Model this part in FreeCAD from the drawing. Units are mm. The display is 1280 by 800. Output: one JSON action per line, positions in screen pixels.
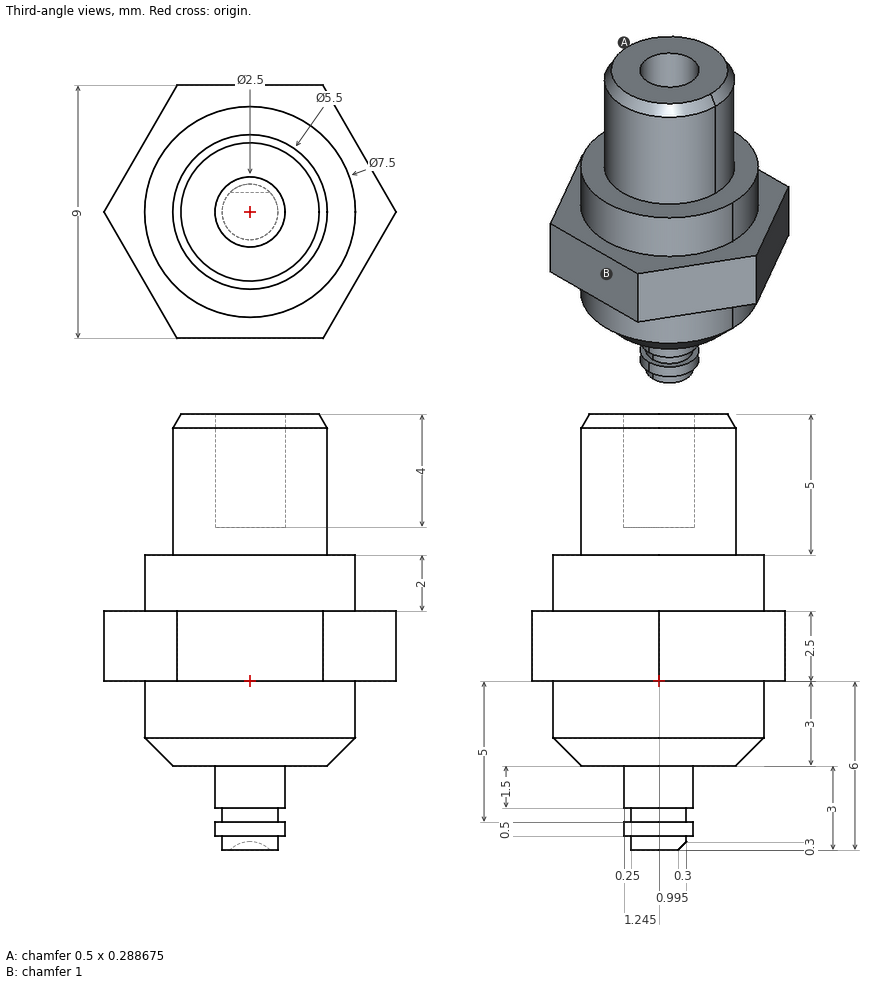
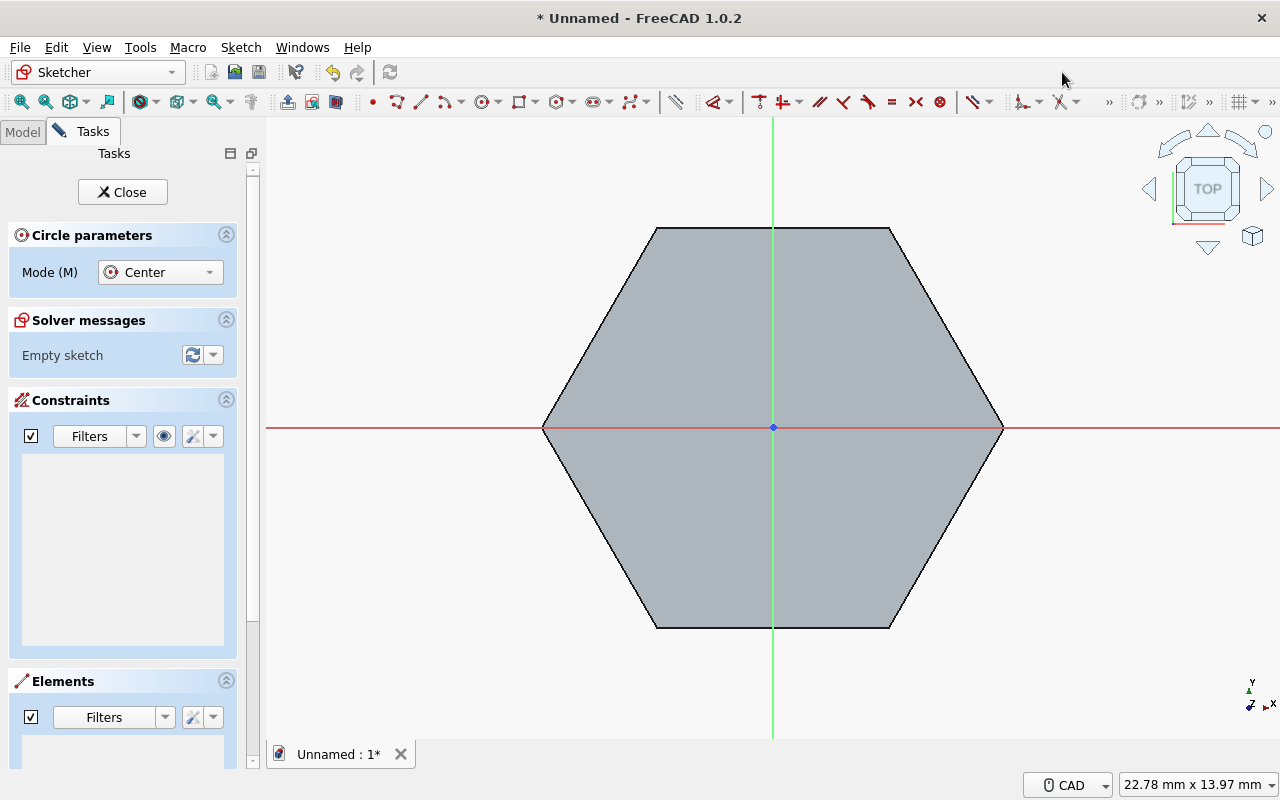
{"action": "left_click", "coordinate": [773, 428]}
{"action": "left_click", "coordinate": [891, 310]}
{"action": "key", "text": "Escape"}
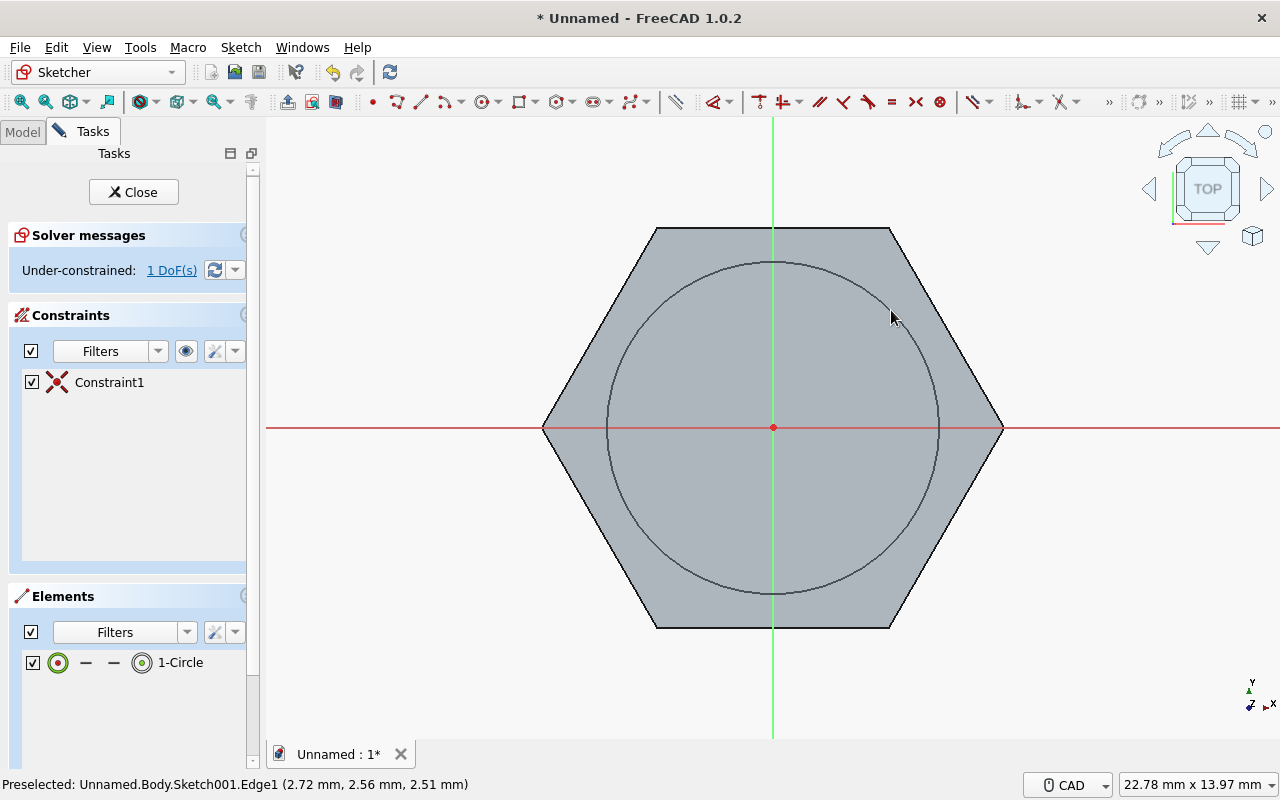
{"action": "left_click", "coordinate": [890, 310]}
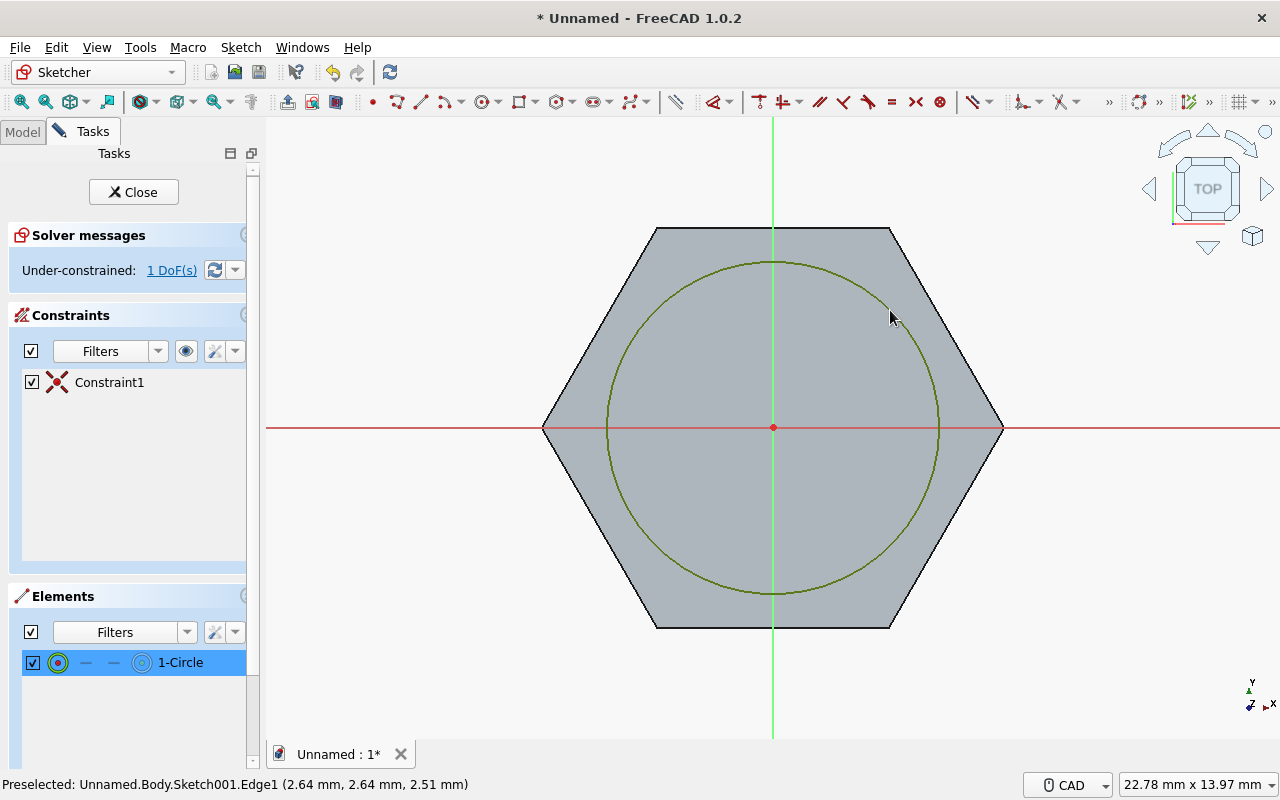
{"action": "key", "text": "k o"}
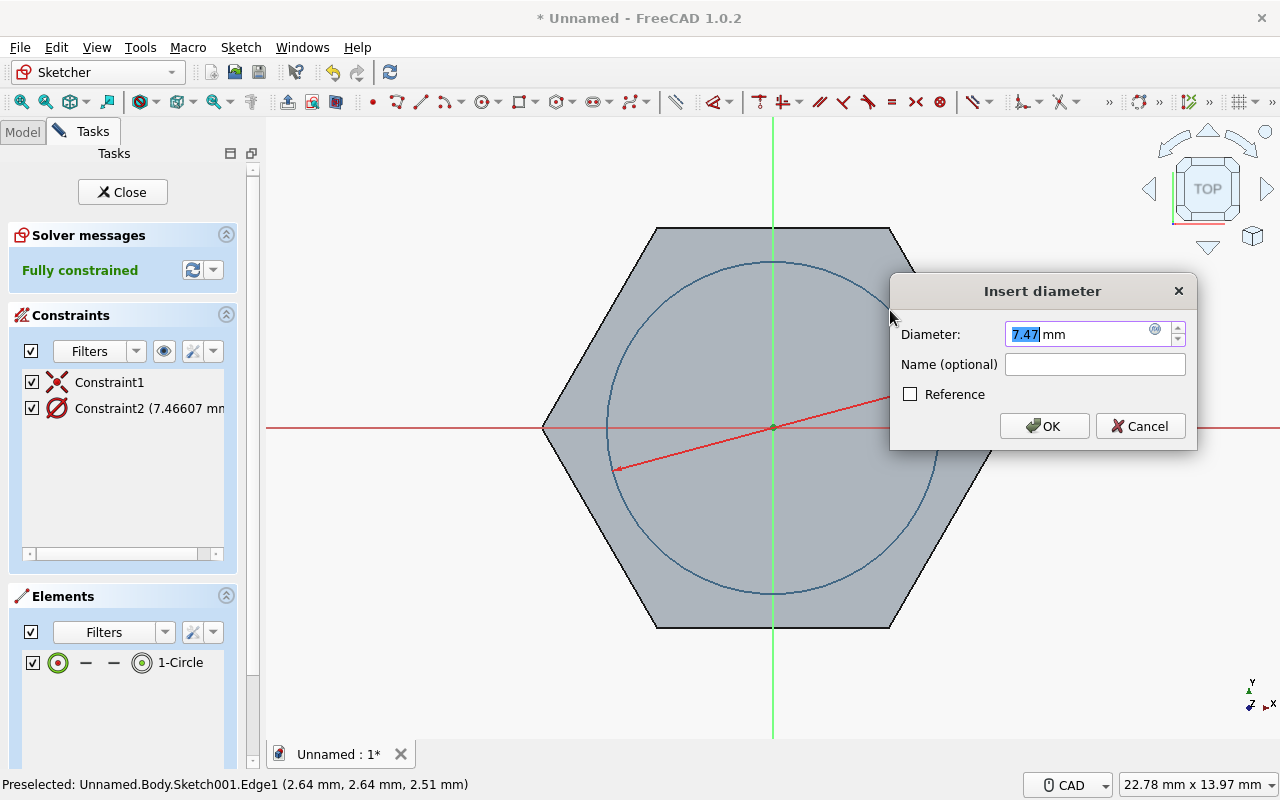
{"action": "type", "text": "7.5"}
{"action": "key", "text": "Return"}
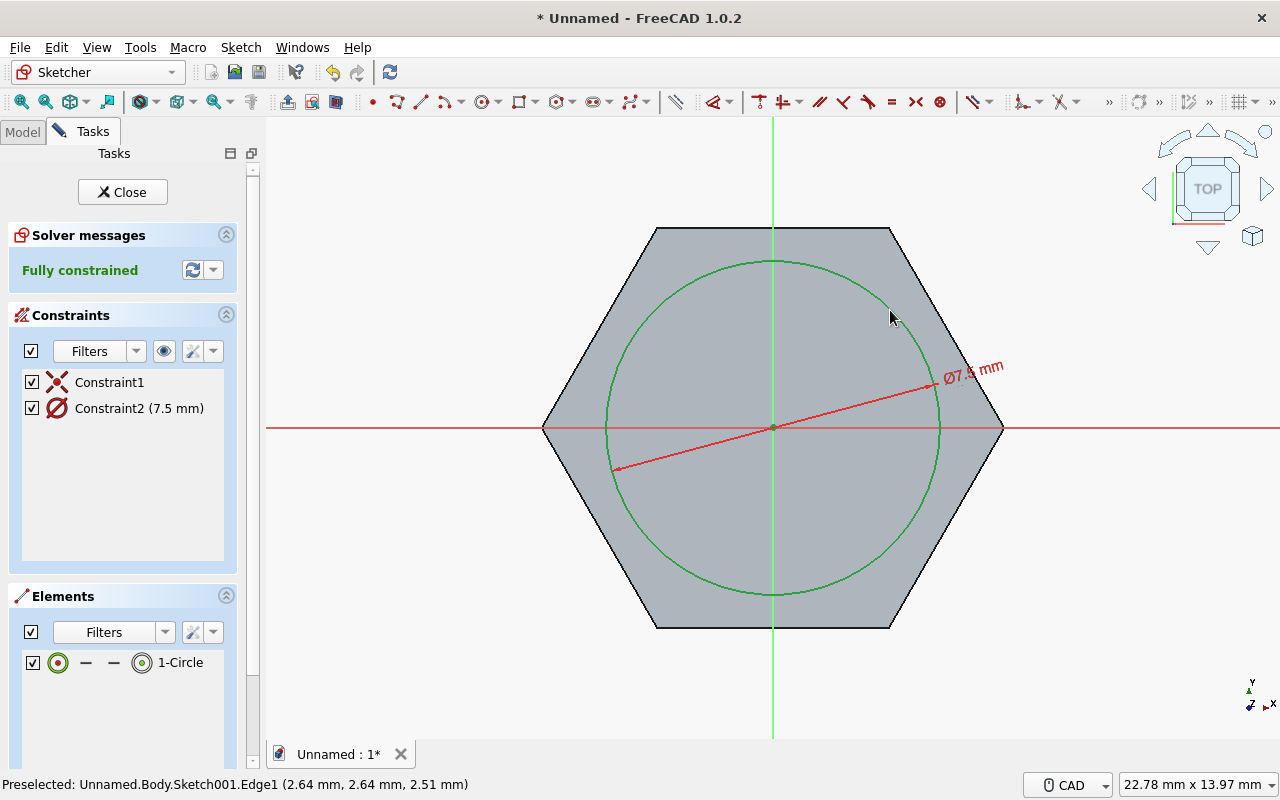
{"action": "left_click", "coordinate": [123, 192]}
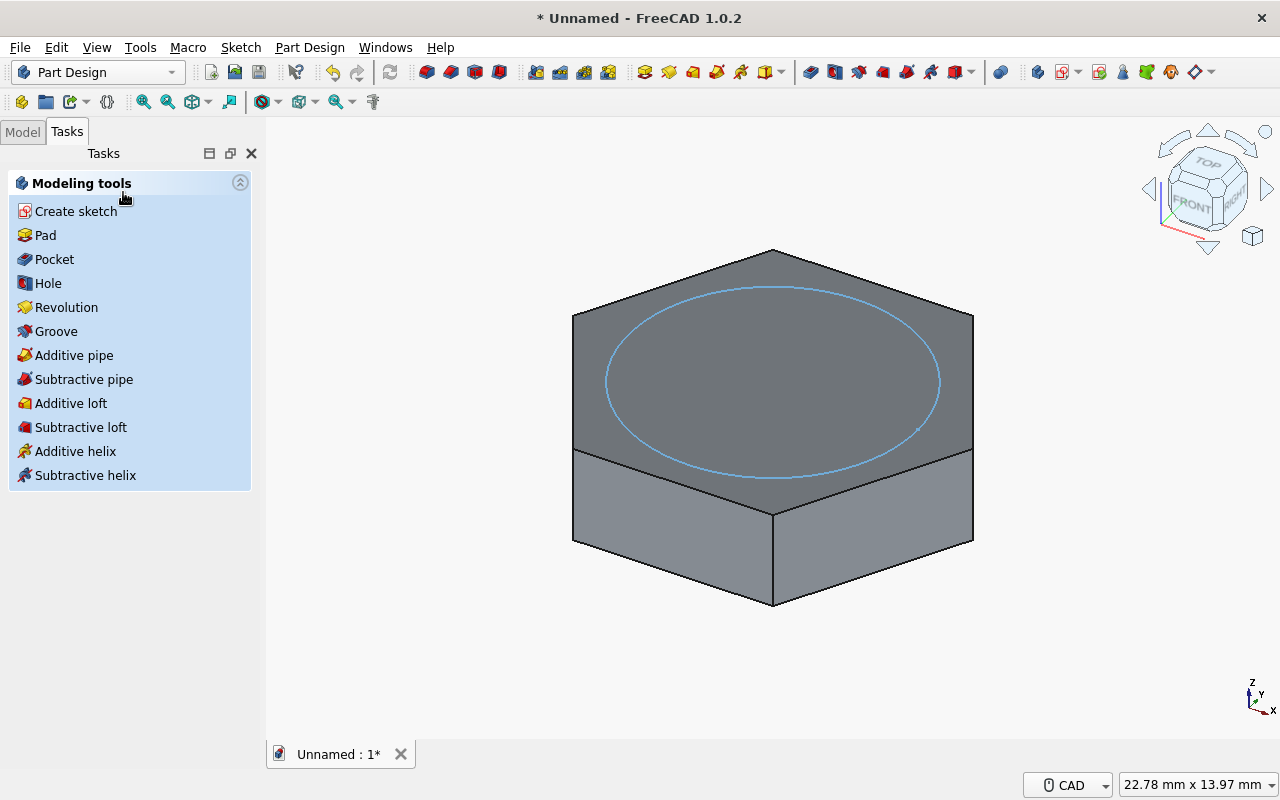
{"action": "left_click", "coordinate": [646, 72]}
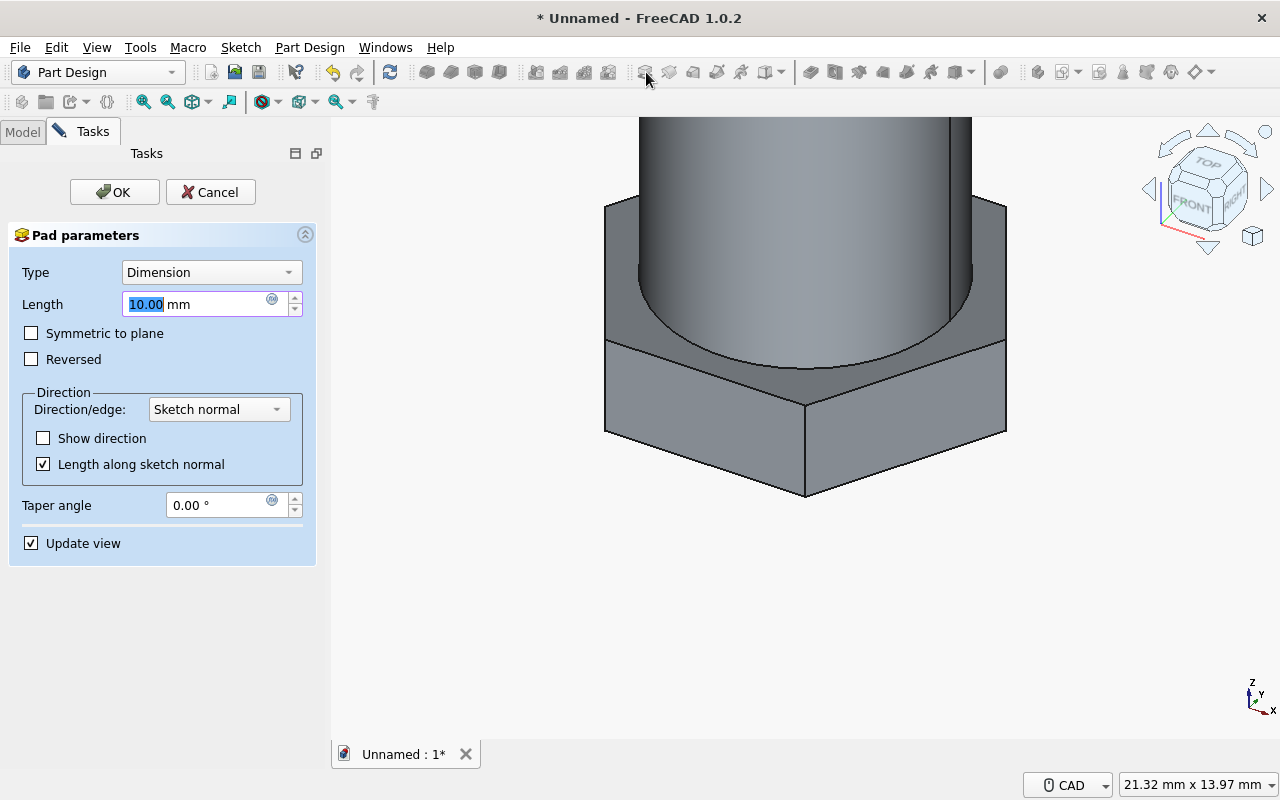
{"action": "type", "text": "2"}
{"action": "key", "text": "Tab"}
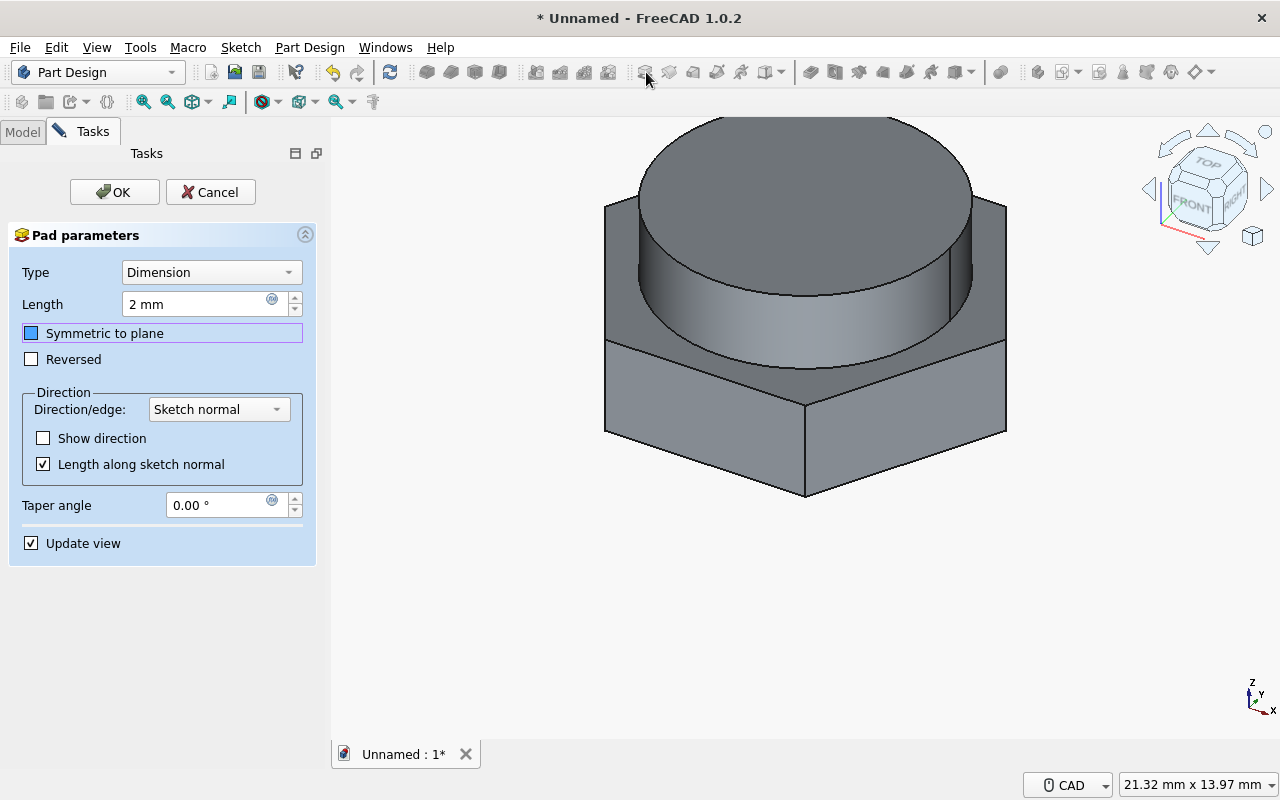
{"action": "left_click", "coordinate": [115, 192]}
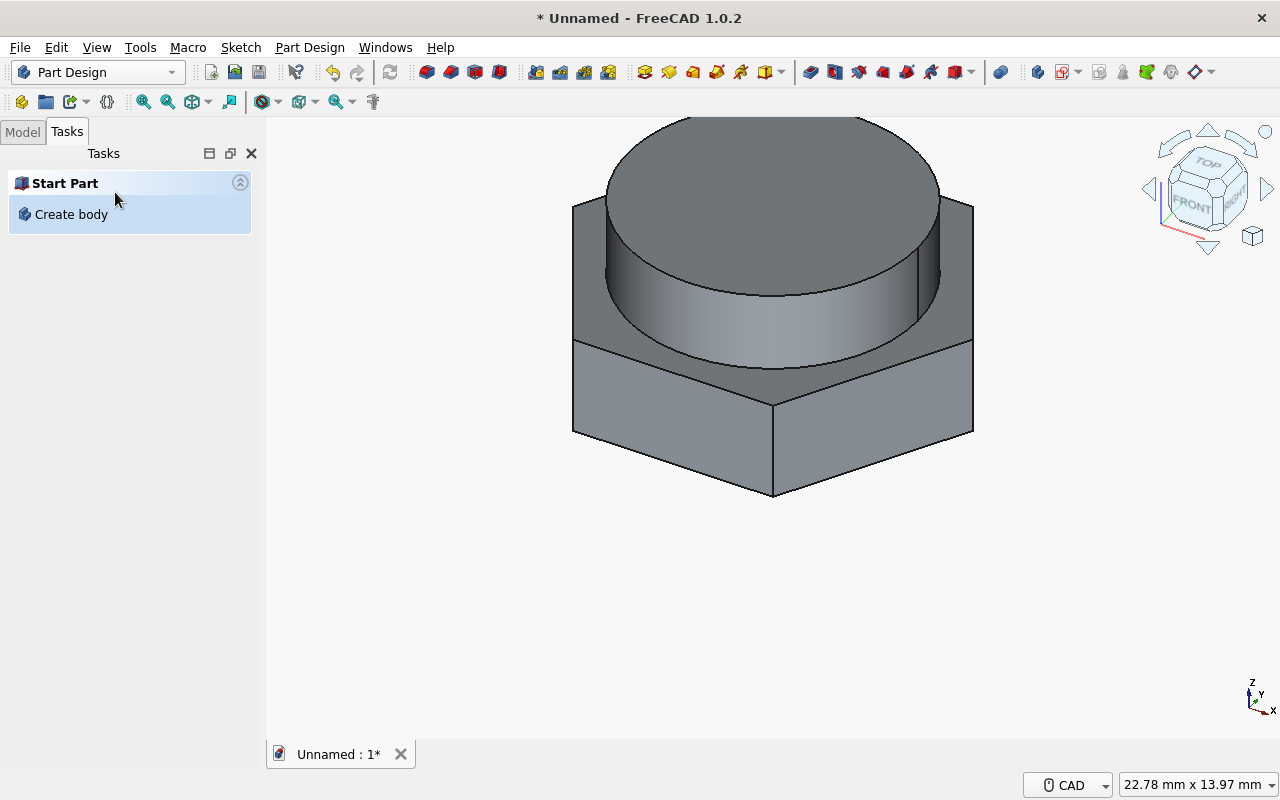
{"action": "key", "text": "v f"}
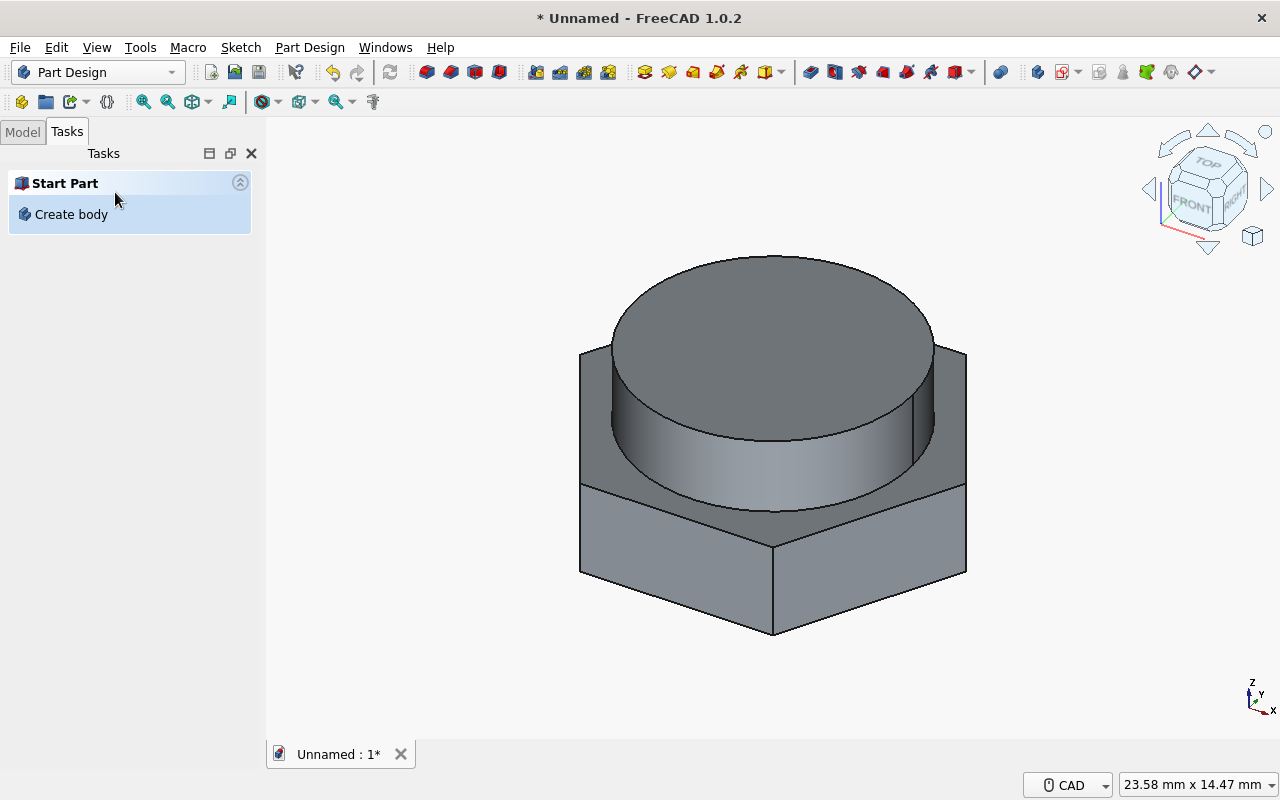
{"action": "left_click", "coordinate": [773, 348]}